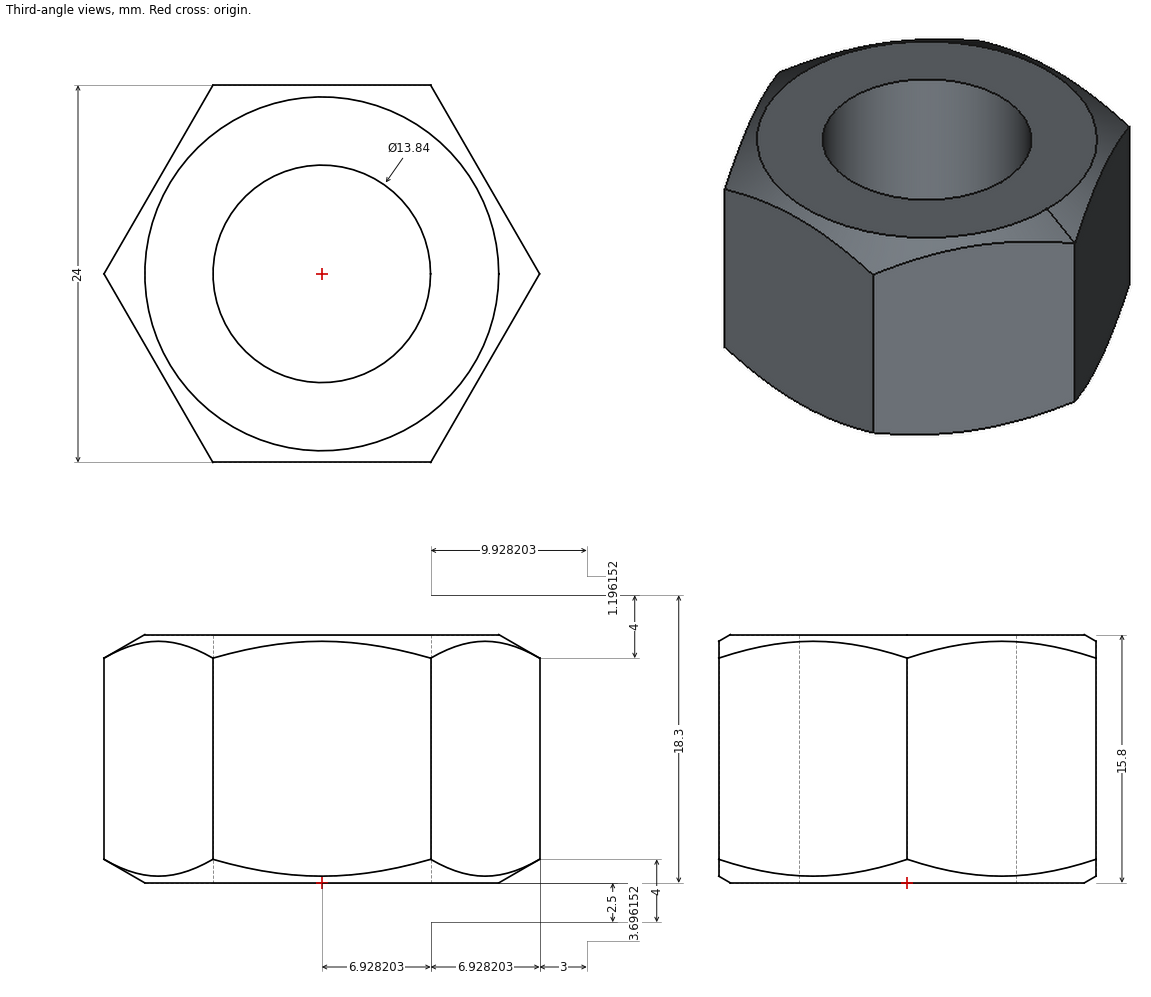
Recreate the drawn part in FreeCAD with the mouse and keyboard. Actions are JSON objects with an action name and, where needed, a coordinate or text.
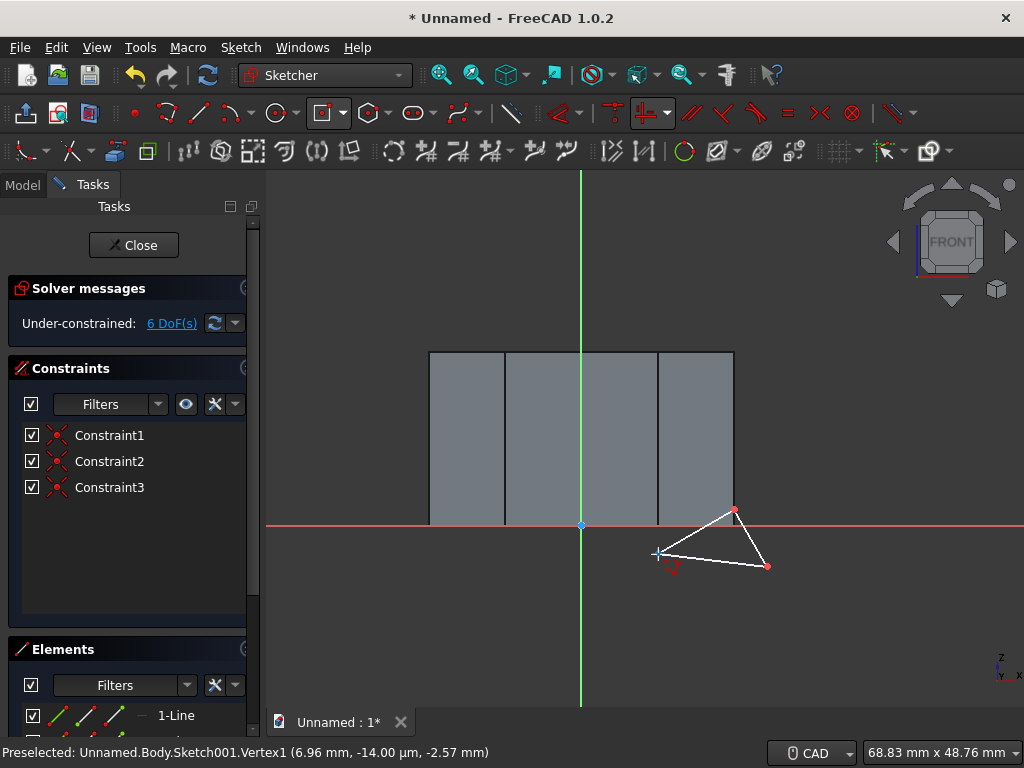
{"action": "left_click", "coordinate": [658, 324]}
{"action": "left_click", "coordinate": [767, 311]}
{"action": "left_click", "coordinate": [734, 368]}
{"action": "left_click", "coordinate": [658, 325]}
{"action": "key", "text": "Escape"}
{"action": "key", "text": "Escape"}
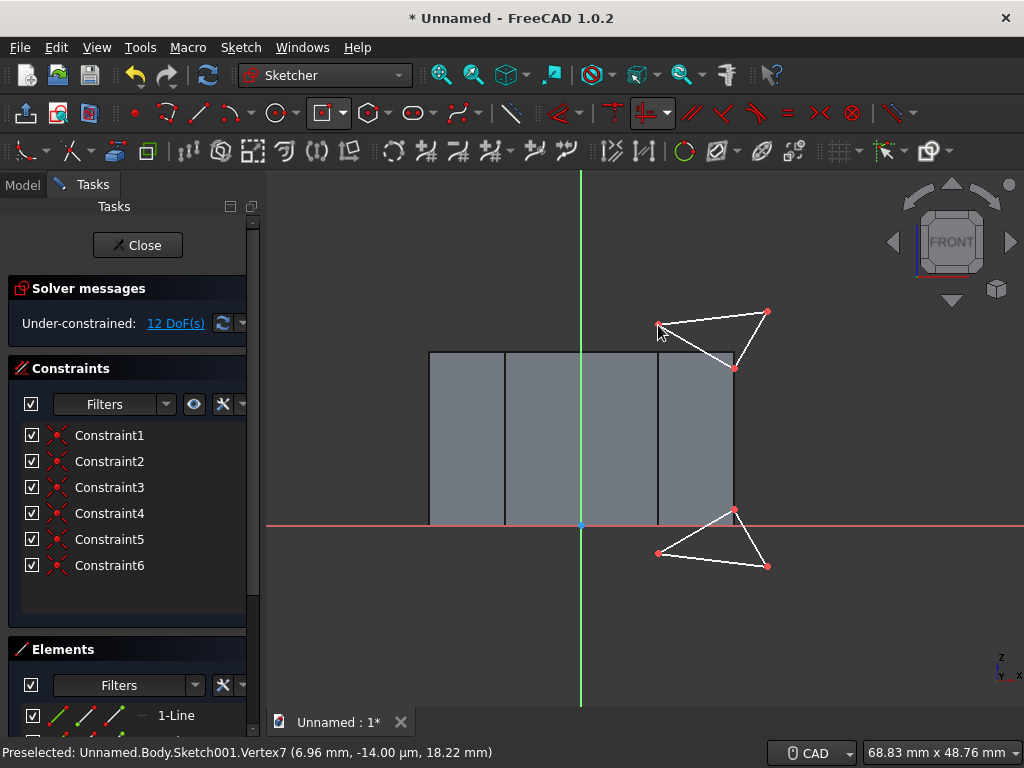
{"action": "left_click", "coordinate": [558, 114]}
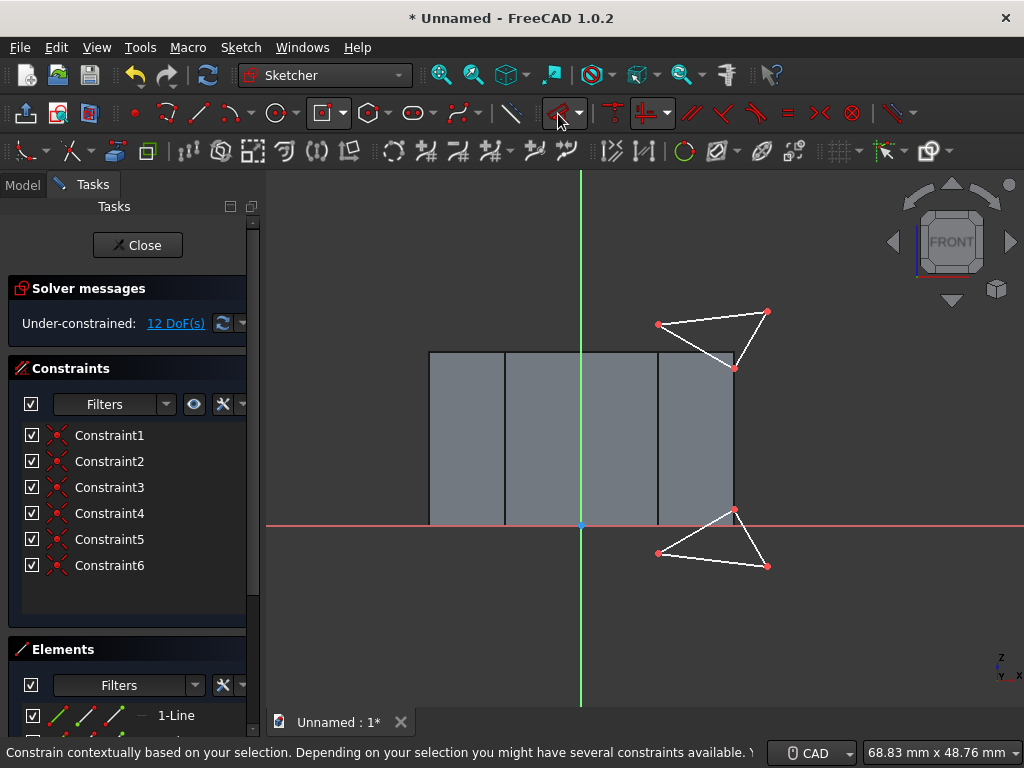
{"action": "left_click", "coordinate": [681, 541]}
{"action": "left_click", "coordinate": [768, 542]}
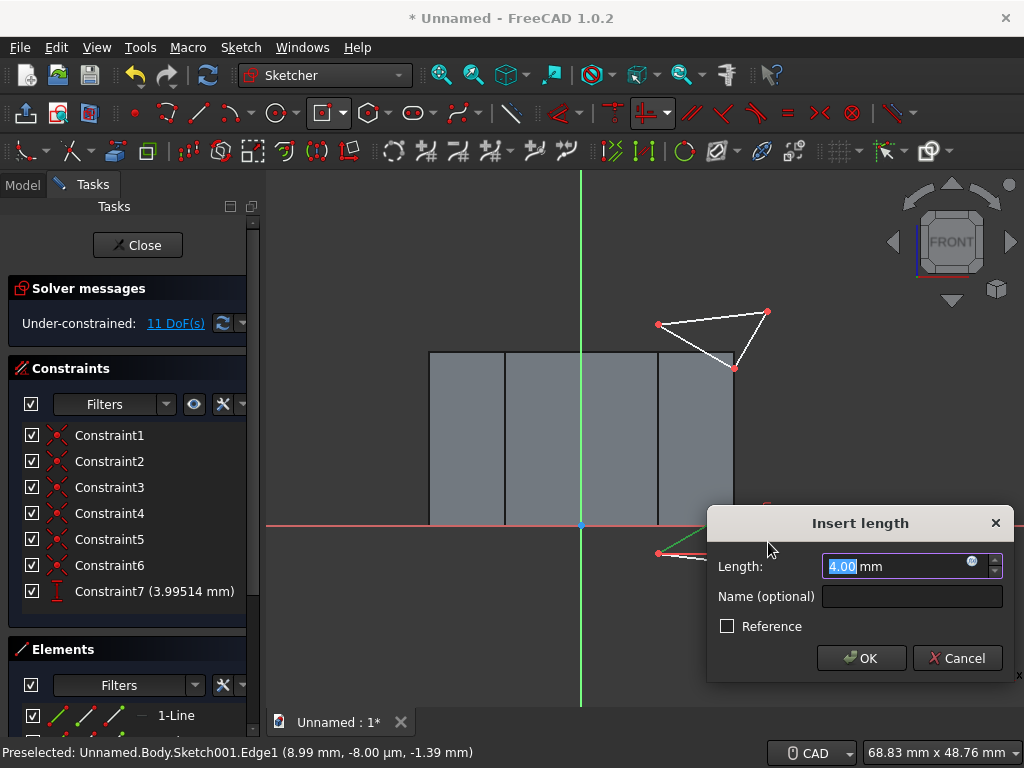
{"action": "type", "text": "4"}
{"action": "key", "text": "Return"}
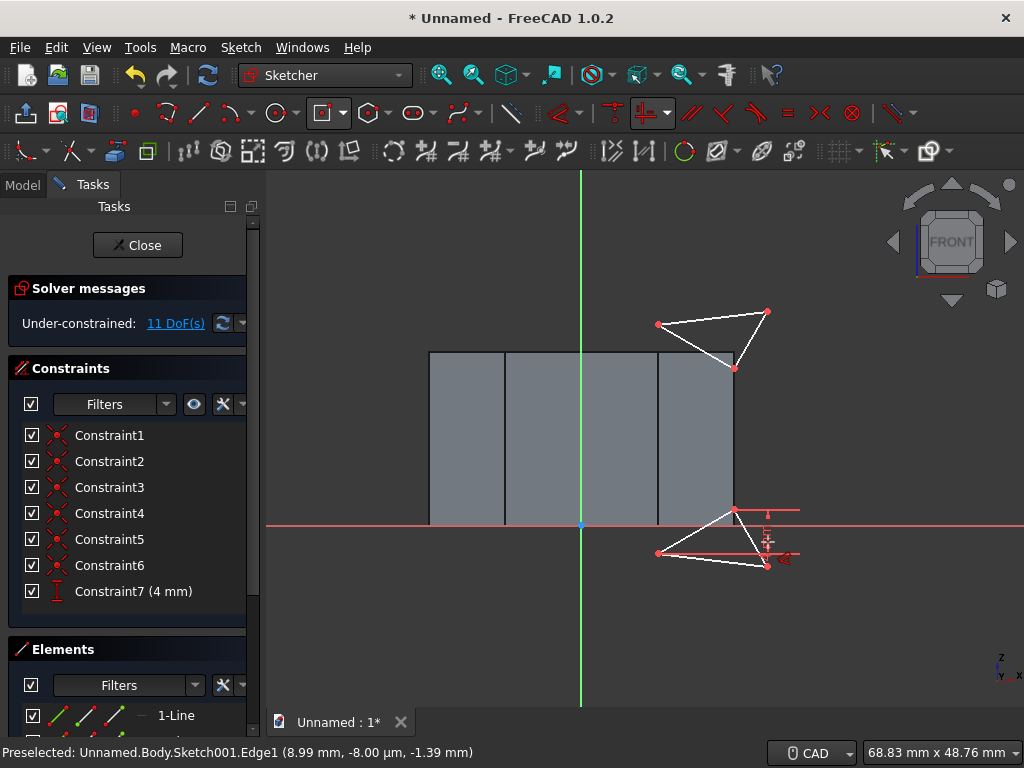
{"action": "left_click", "coordinate": [744, 527]}
{"action": "left_click", "coordinate": [751, 601]}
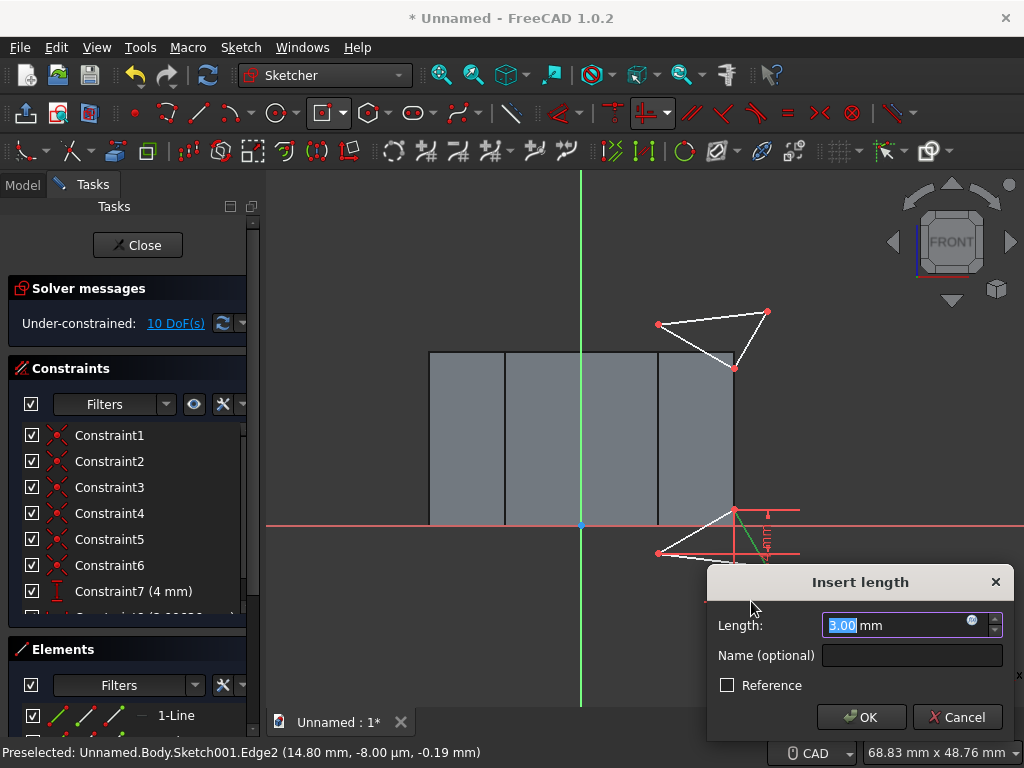
{"action": "type", "text": "3"}
{"action": "key", "text": "Return"}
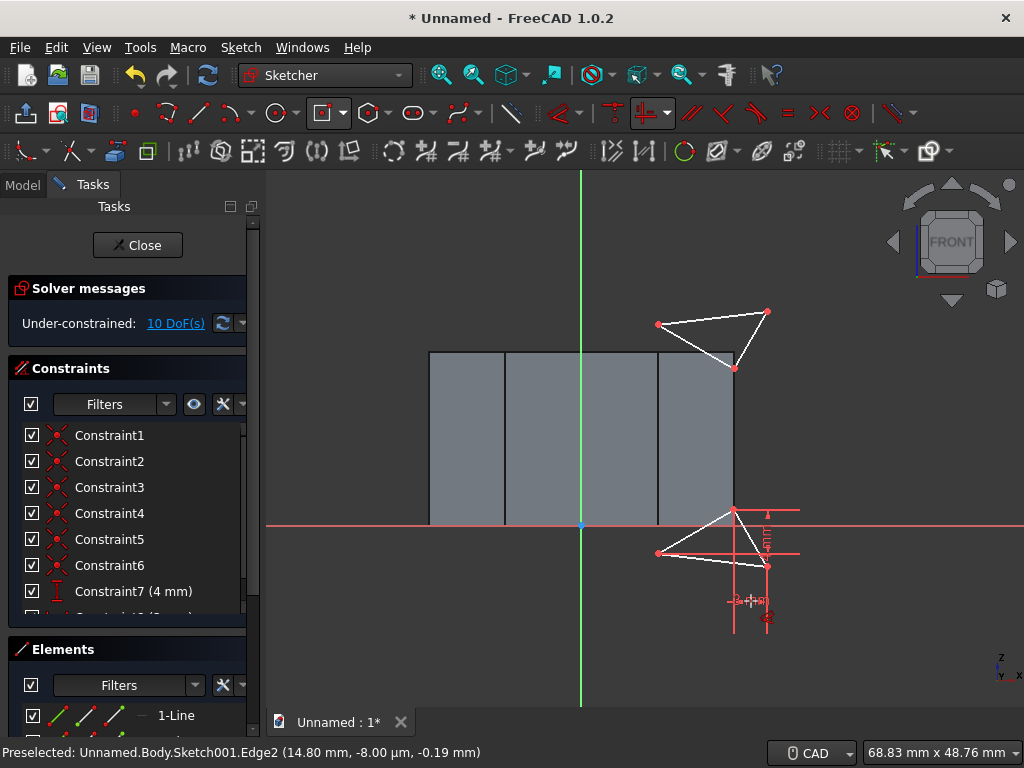
{"action": "left_click", "coordinate": [757, 329]}
{"action": "left_click", "coordinate": [751, 278]}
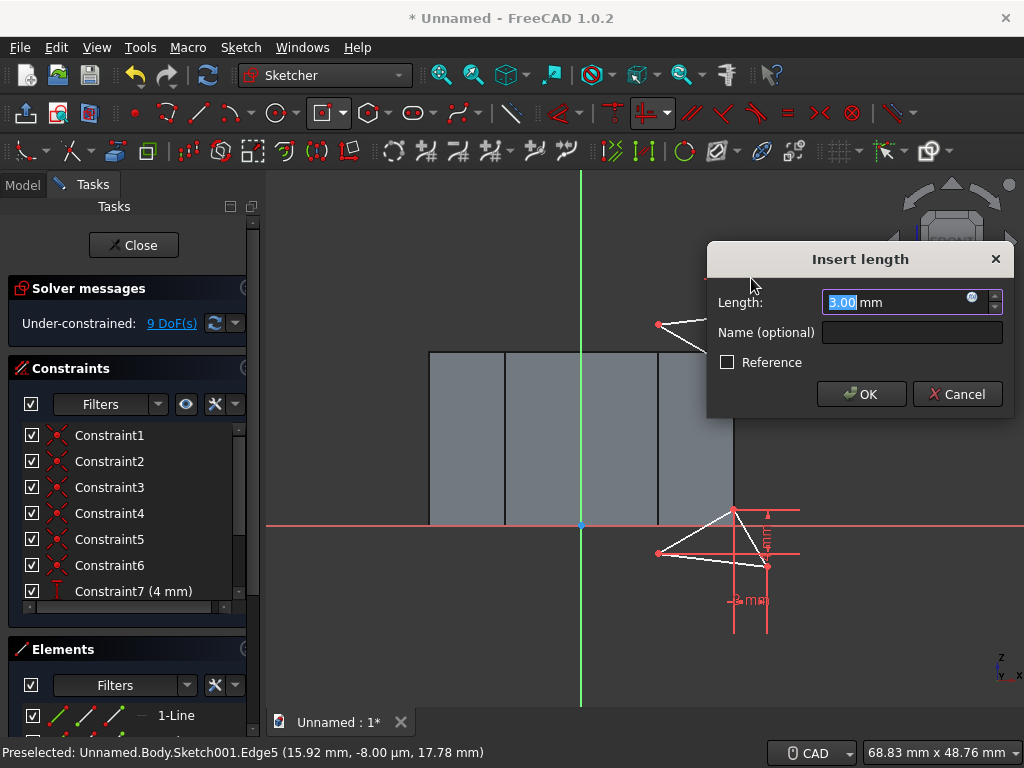
{"action": "type", "text": "3"}
{"action": "key", "text": "Return"}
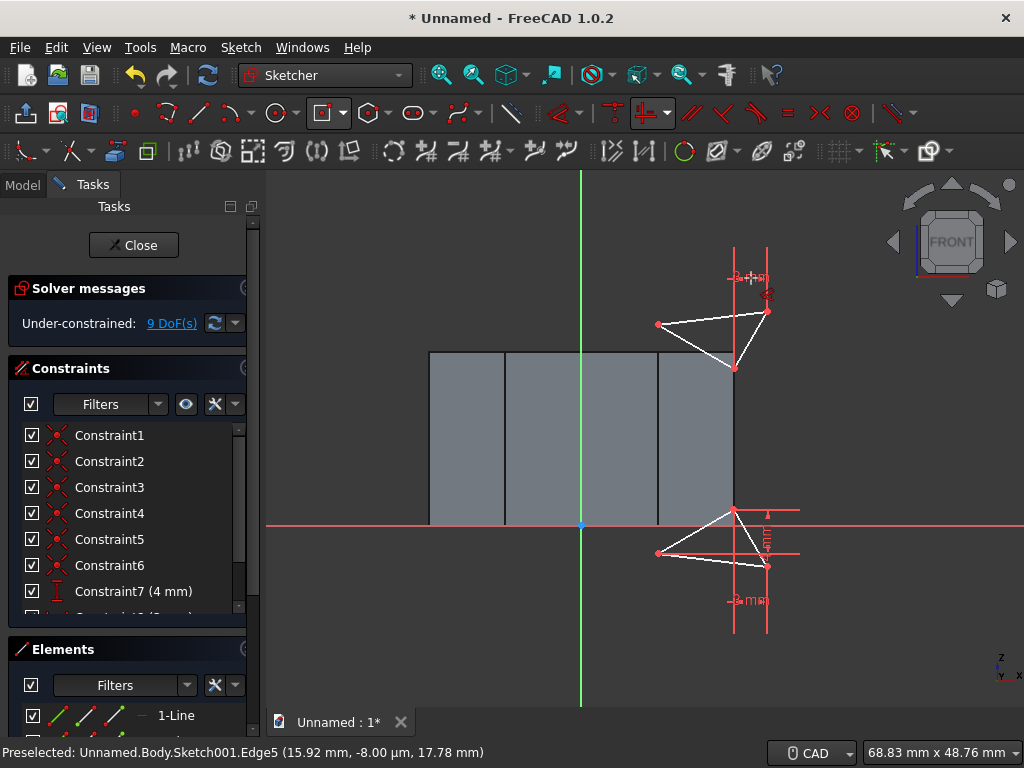
{"action": "left_click", "coordinate": [711, 356]}
{"action": "left_click", "coordinate": [768, 347]}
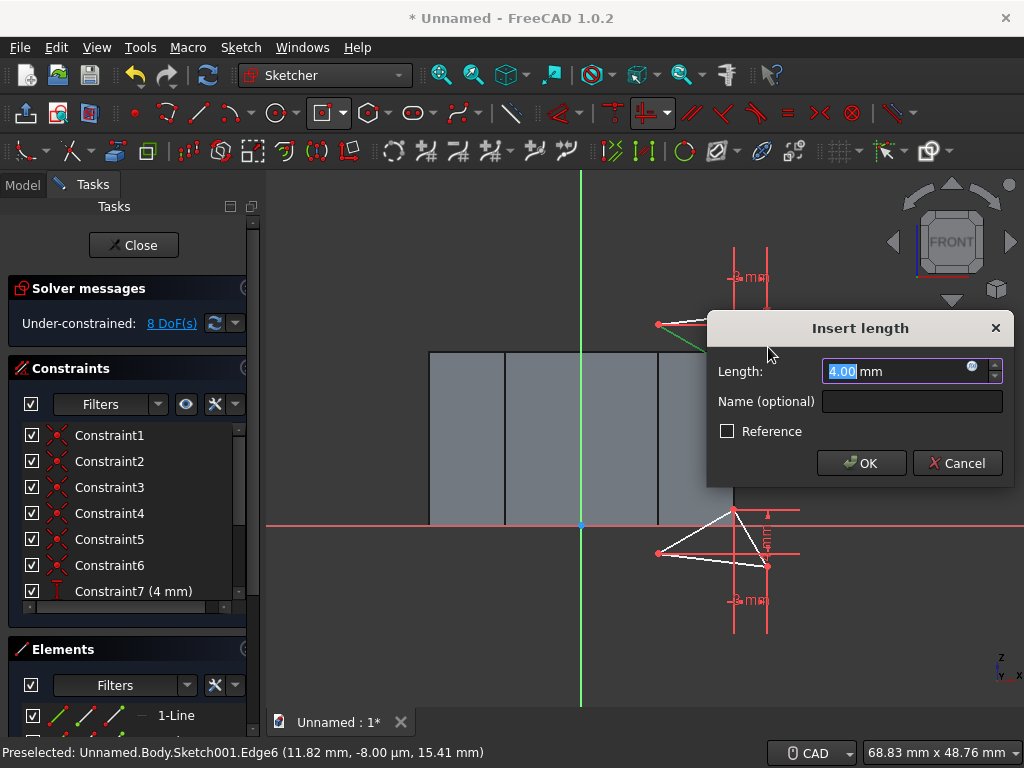
{"action": "type", "text": "4"}
{"action": "key", "text": "Return"}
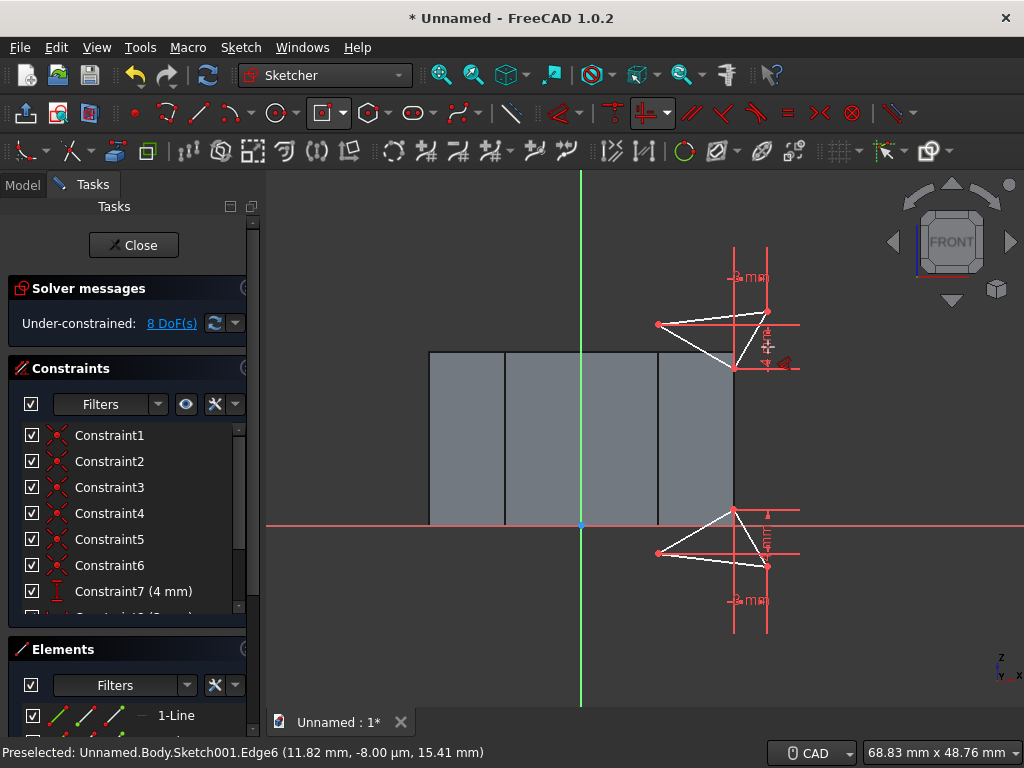
{"action": "scroll", "coordinate": [658, 554], "scroll_direction": "up", "scroll_amount": 2}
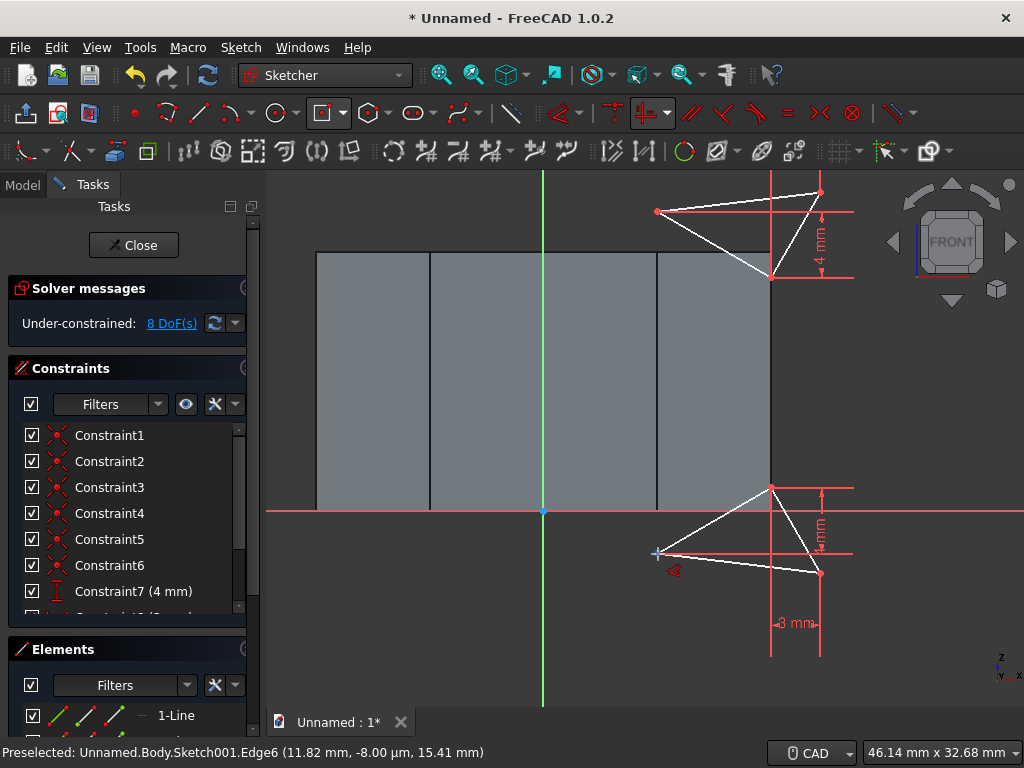
{"action": "left_click", "coordinate": [658, 554]}
{"action": "left_click", "coordinate": [509, 533]}